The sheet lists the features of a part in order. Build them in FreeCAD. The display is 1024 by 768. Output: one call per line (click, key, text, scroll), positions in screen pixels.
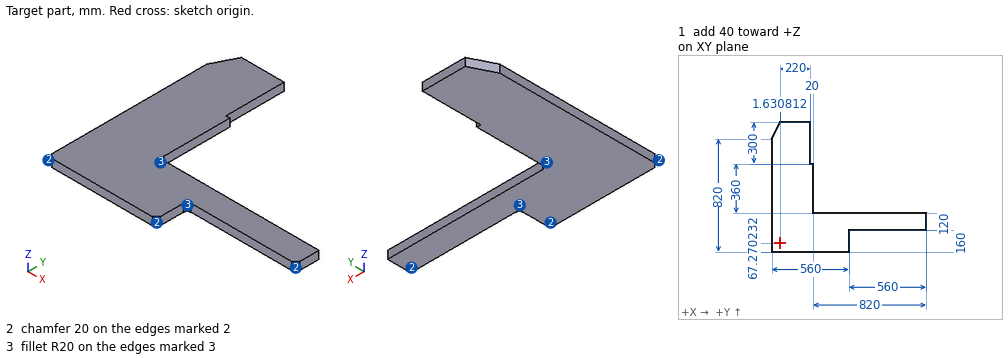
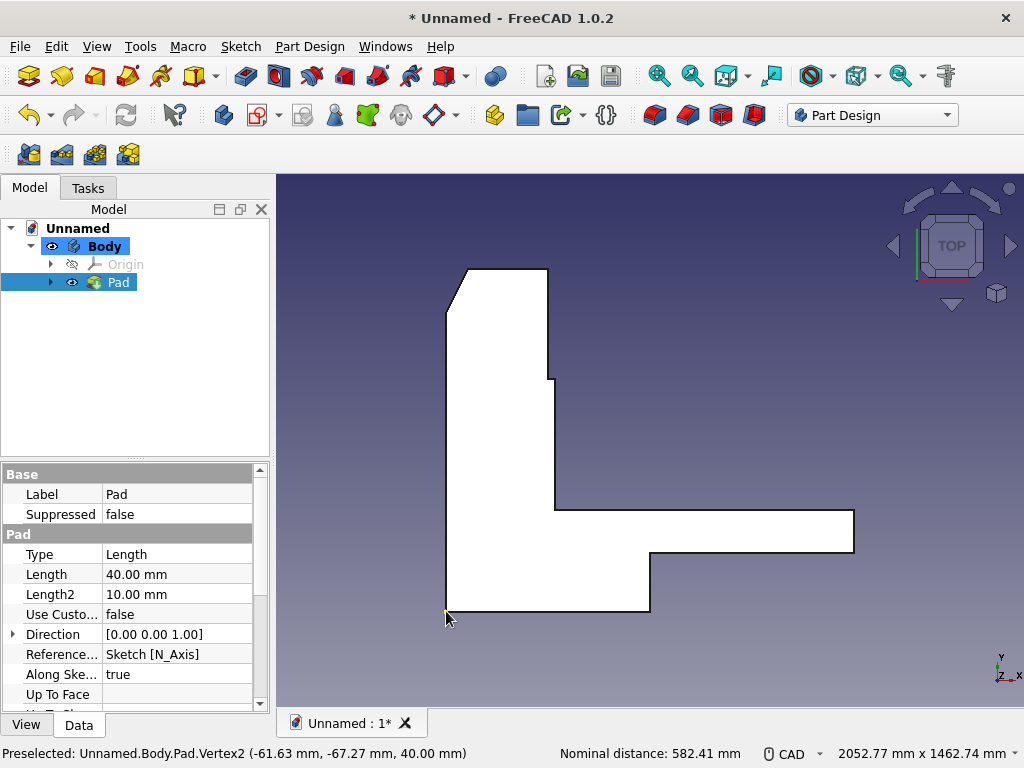
key(1)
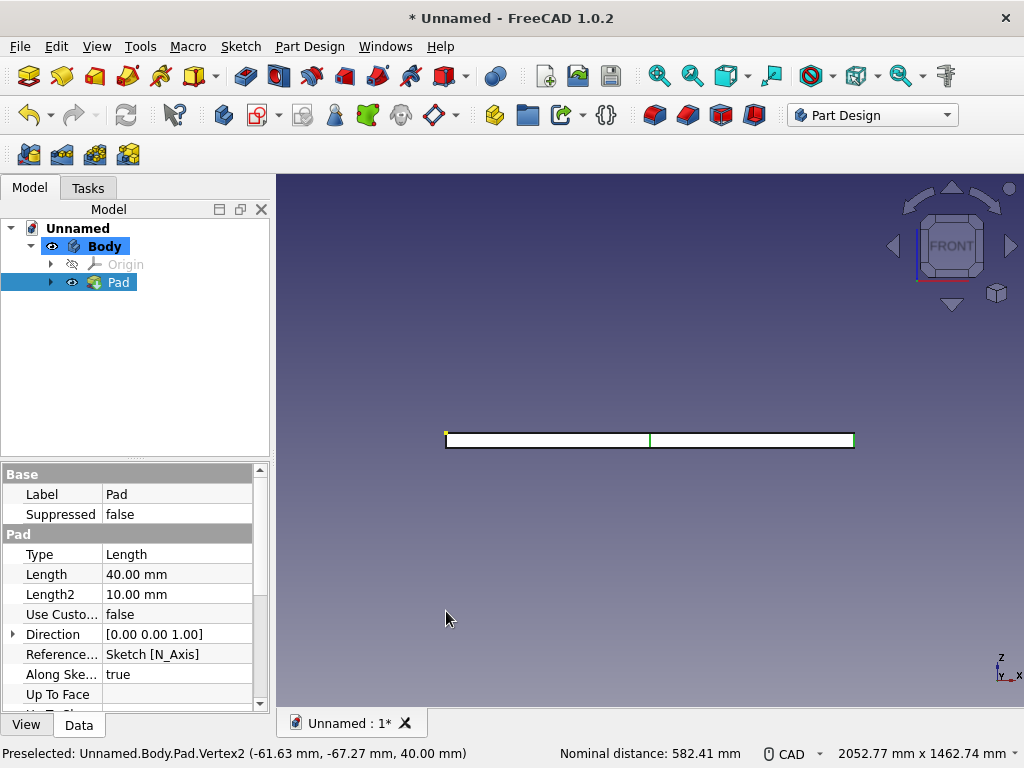
click(446, 439, ctrl)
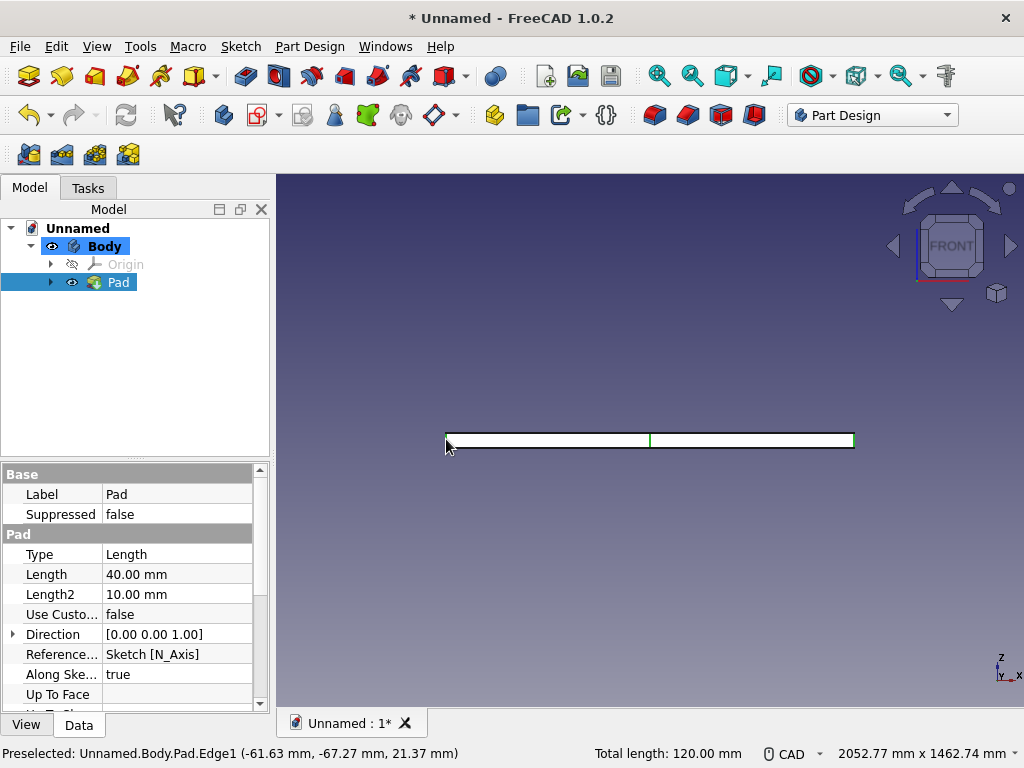
click(688, 116)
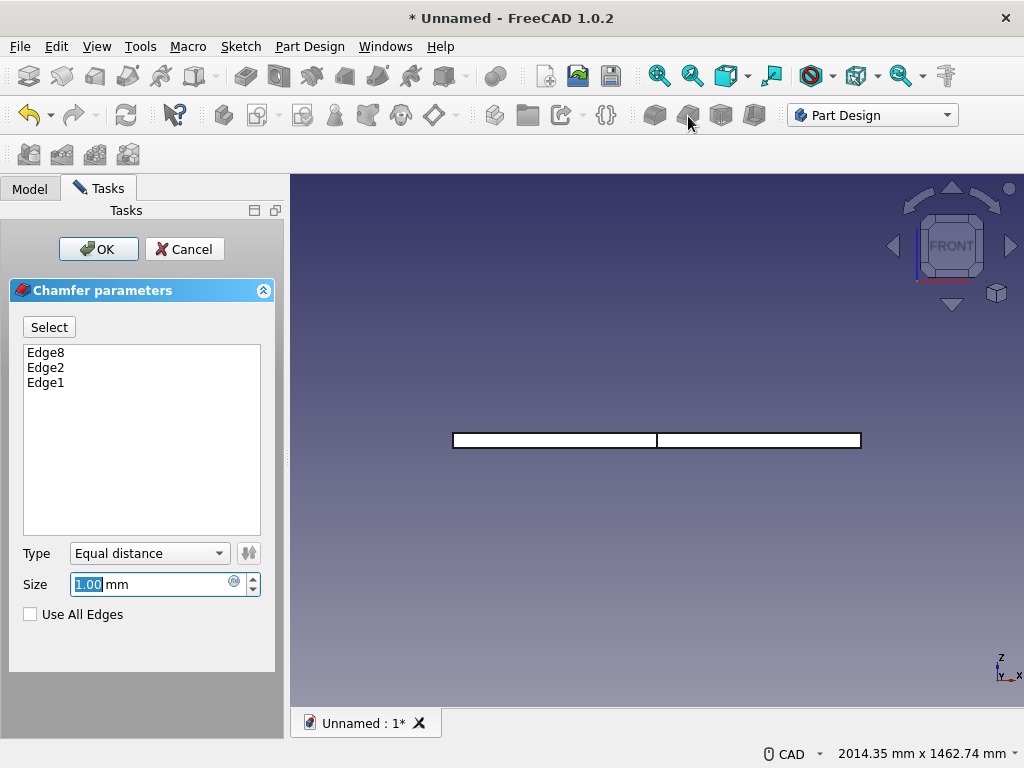
text(20)
key(Tab)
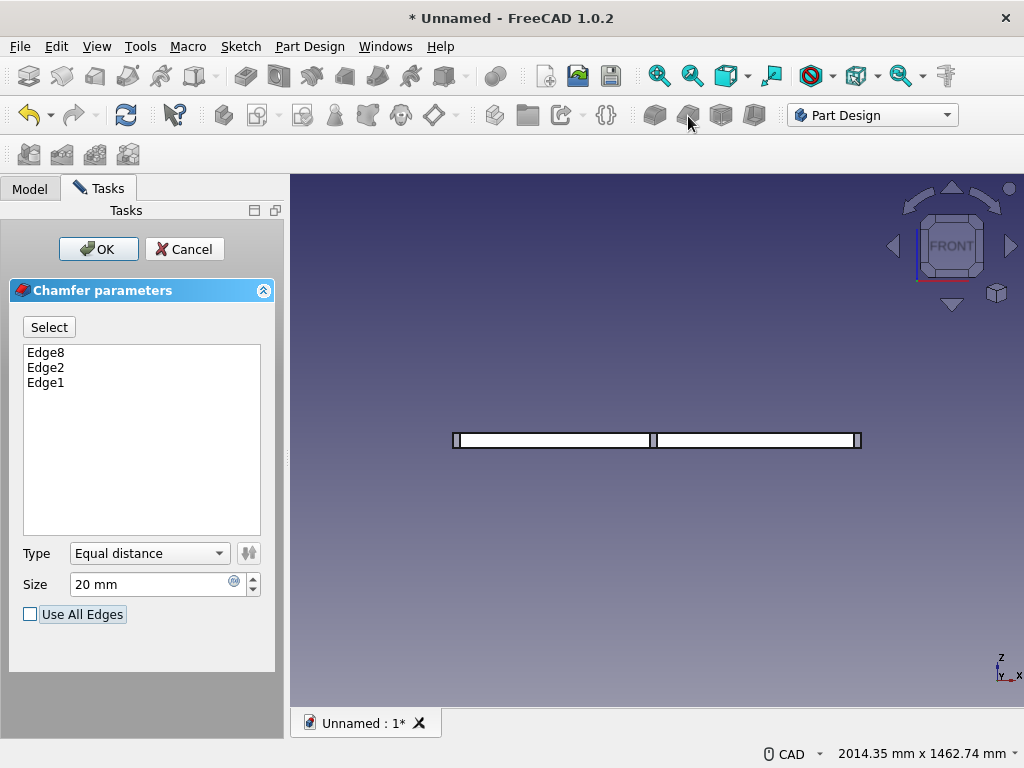
click(99, 249)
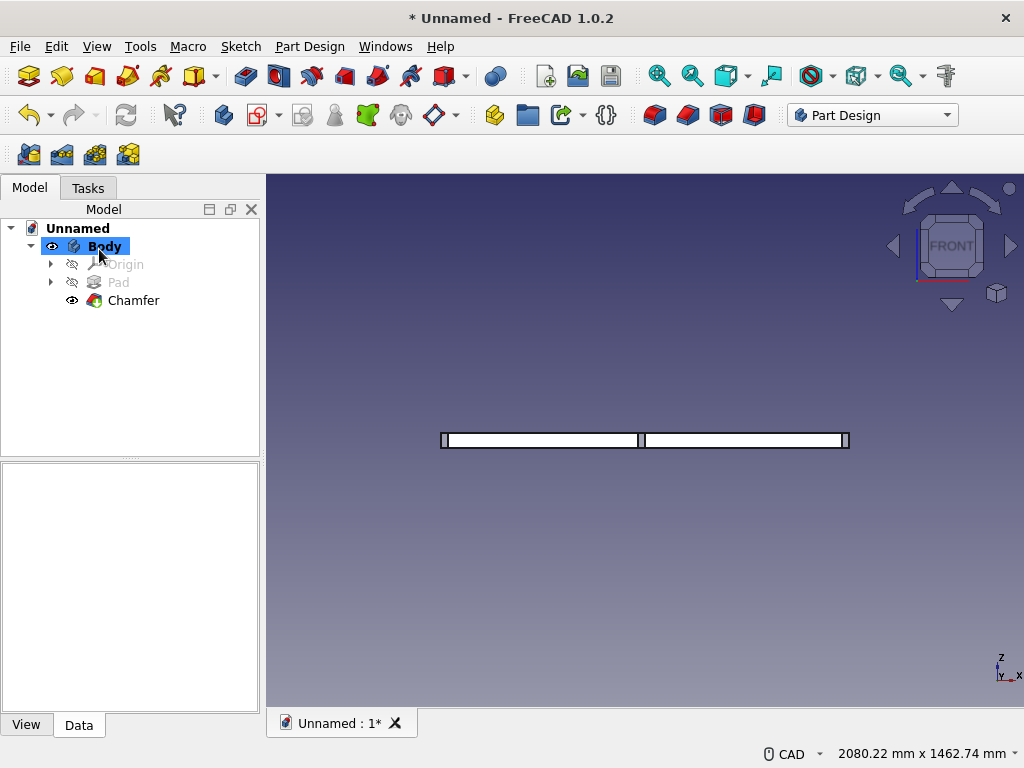
scroll(550, 439, up, 6)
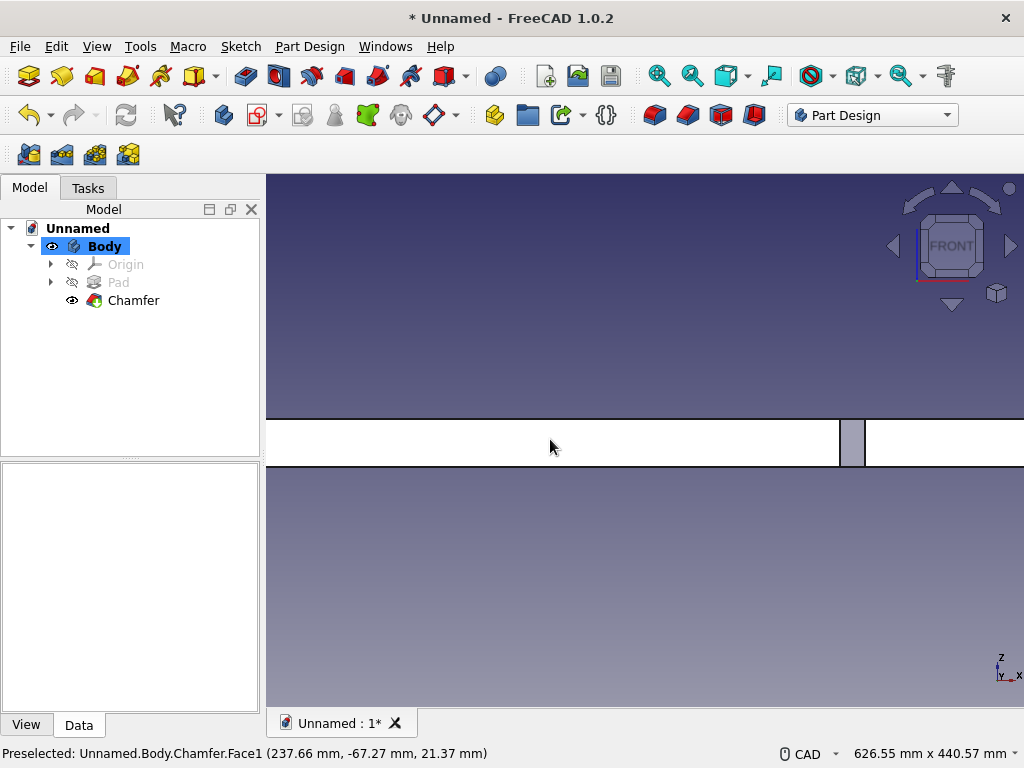
key(v)
key(f)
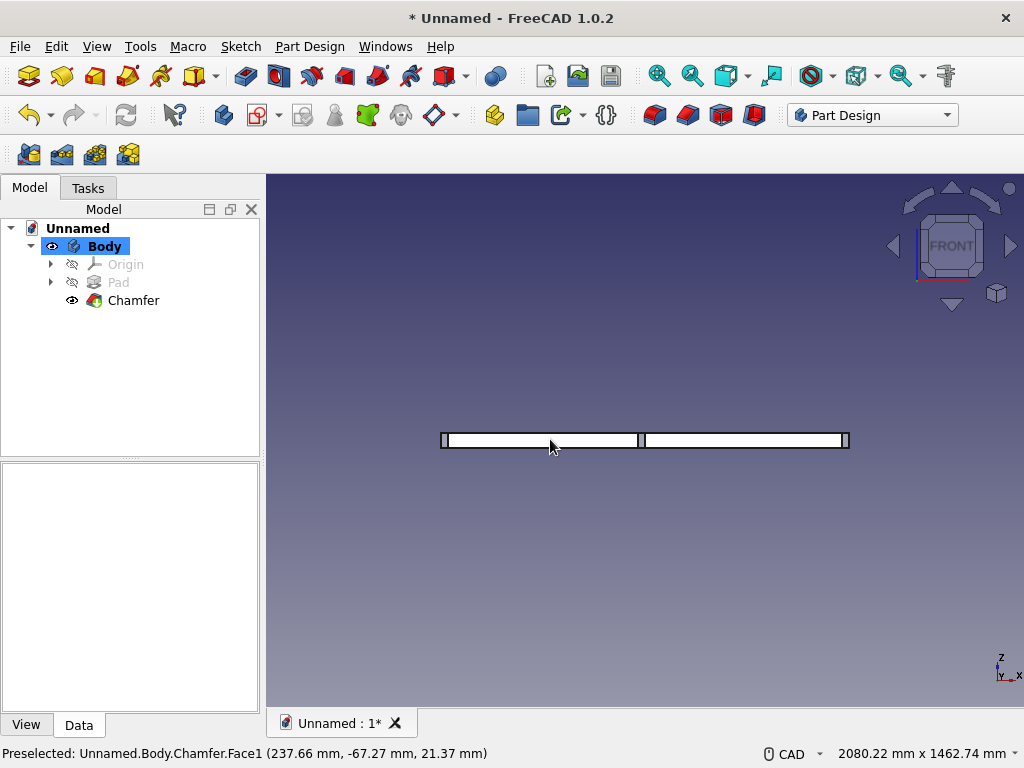
key(0)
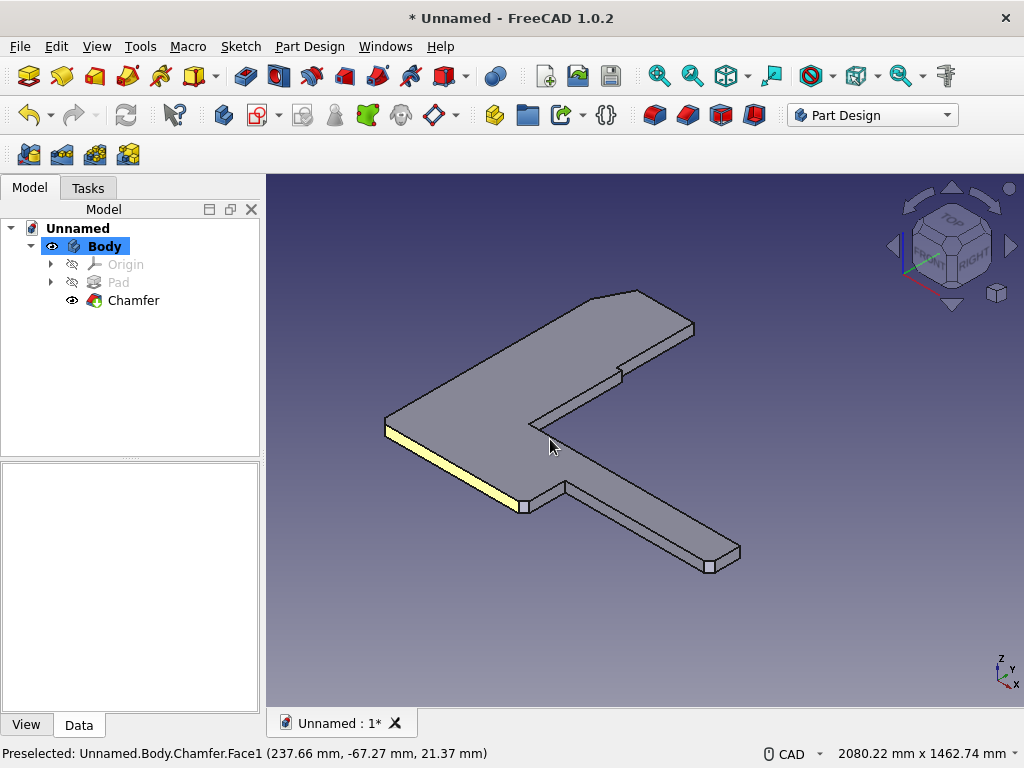
scroll(529, 429, up, 6)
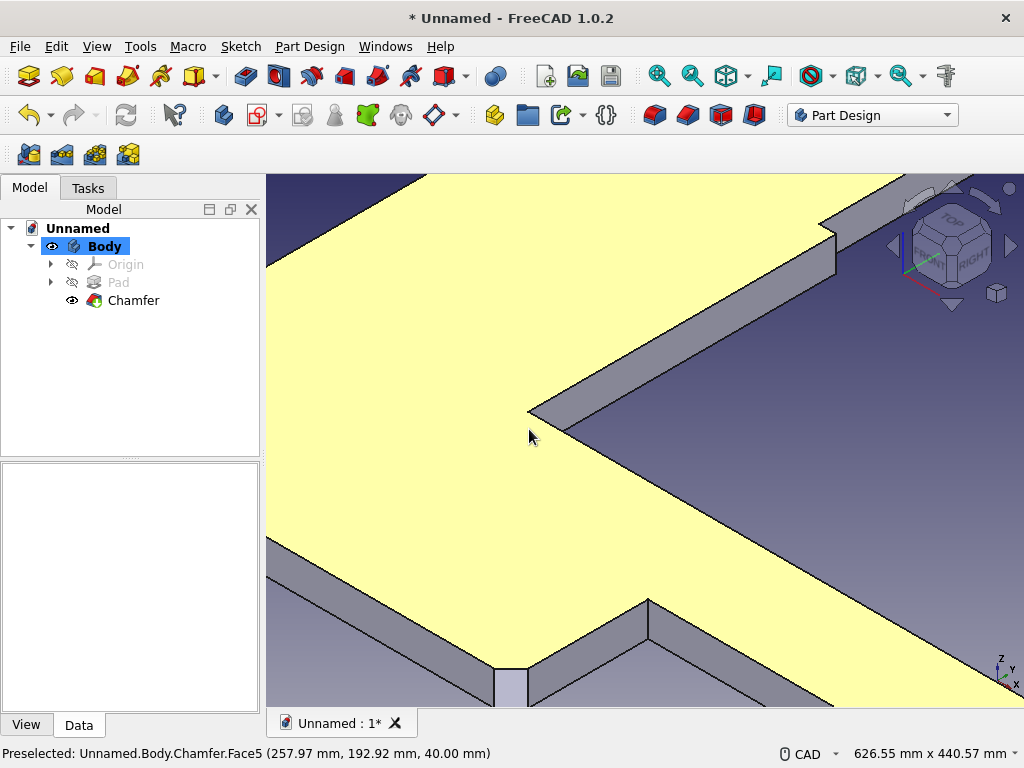
key(v)
key(f)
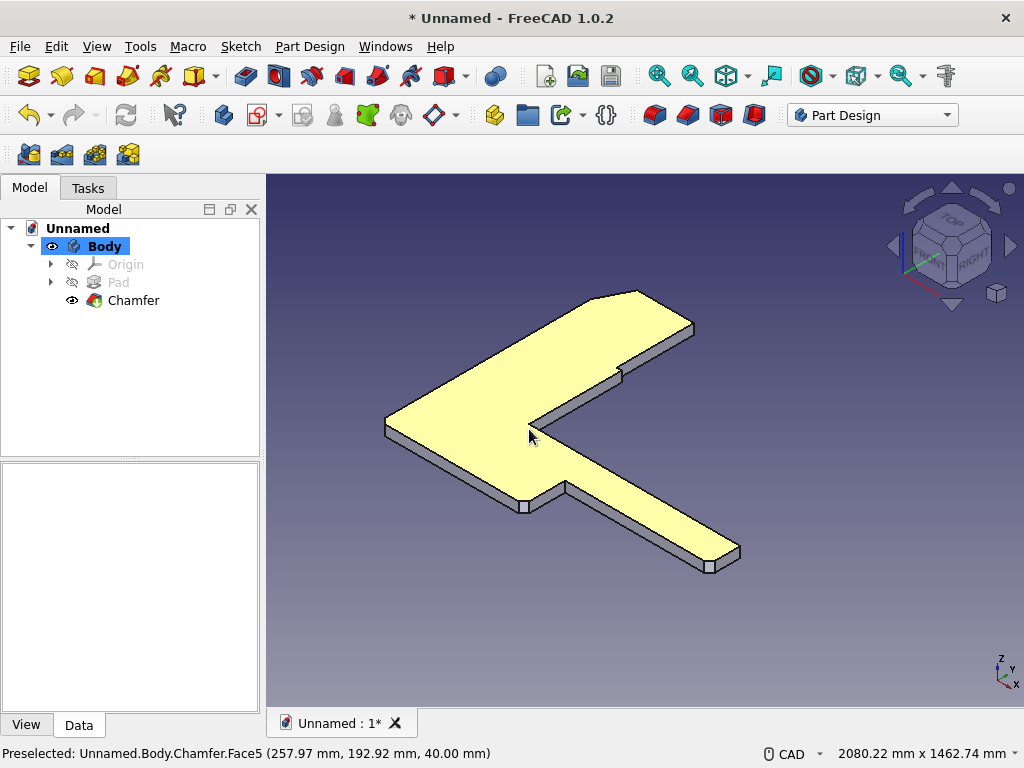
key(2)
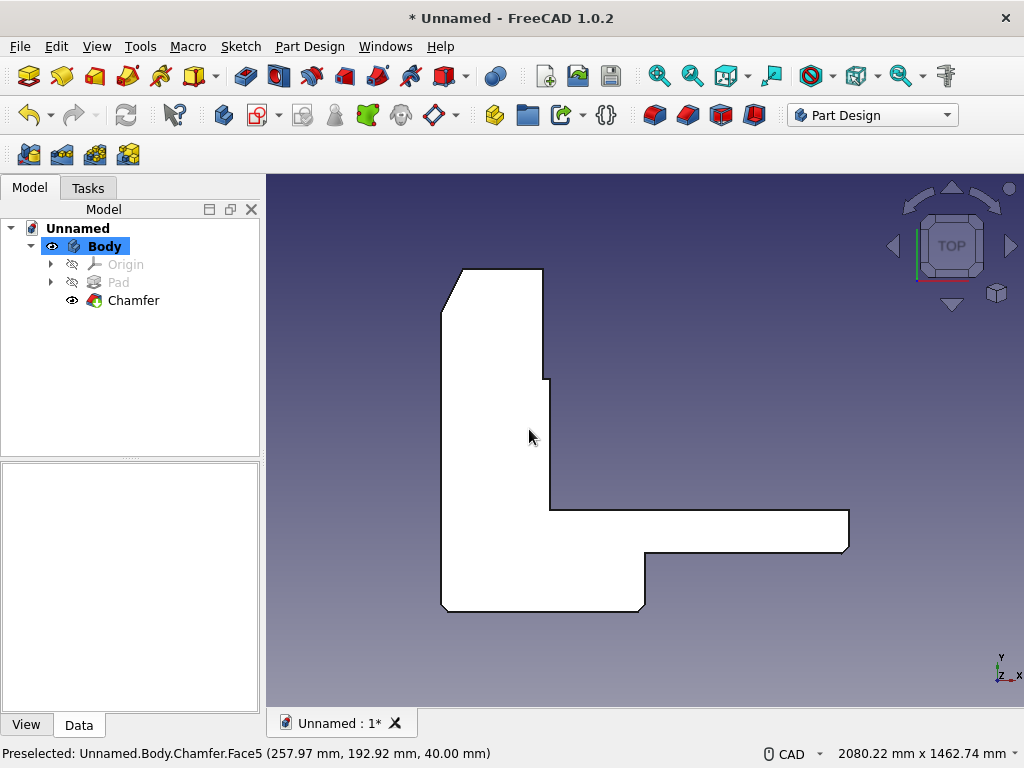
scroll(550, 509, up, 6)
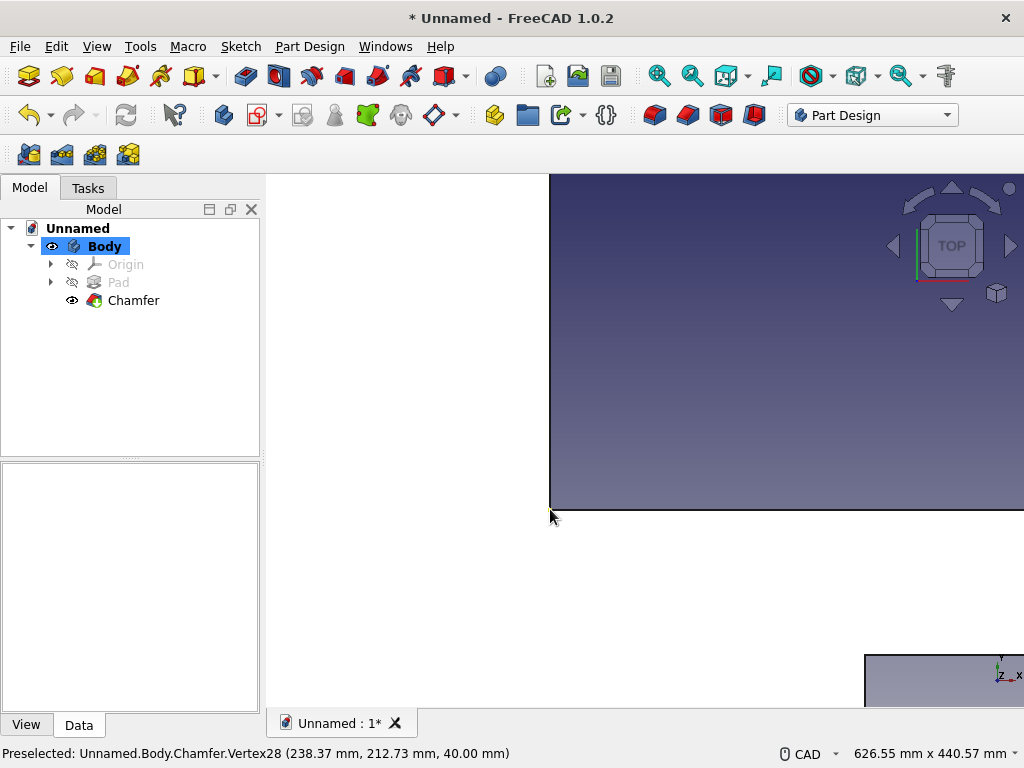
key(v)
key(f)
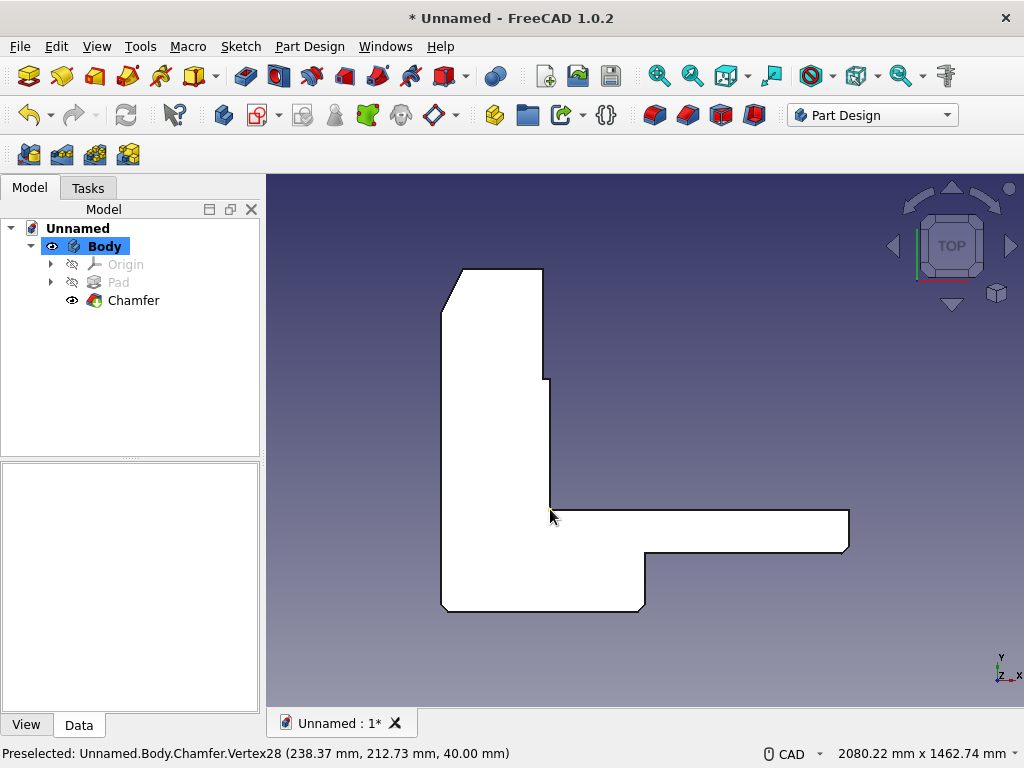
key(1)